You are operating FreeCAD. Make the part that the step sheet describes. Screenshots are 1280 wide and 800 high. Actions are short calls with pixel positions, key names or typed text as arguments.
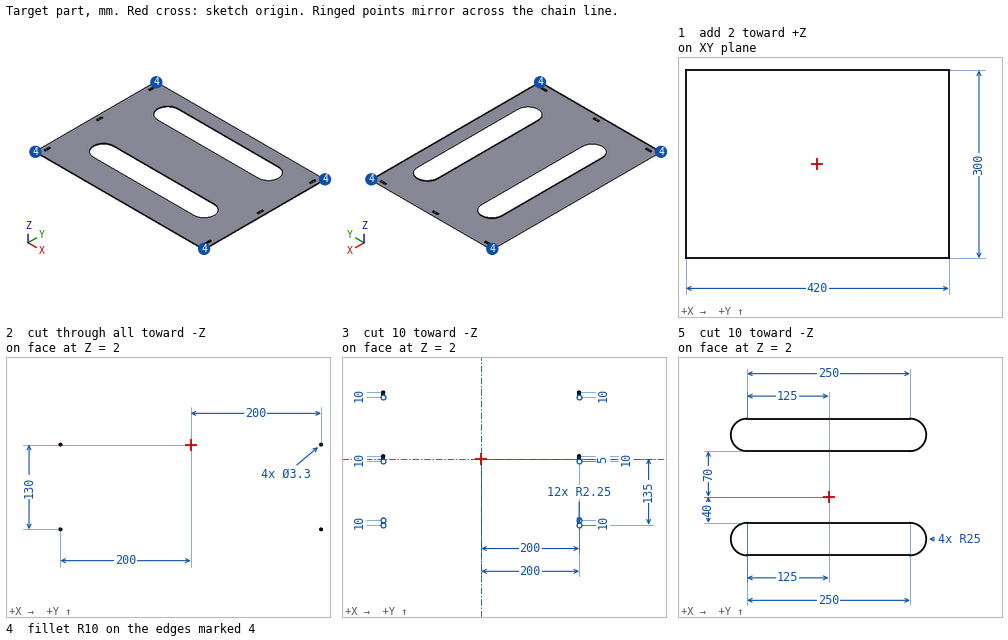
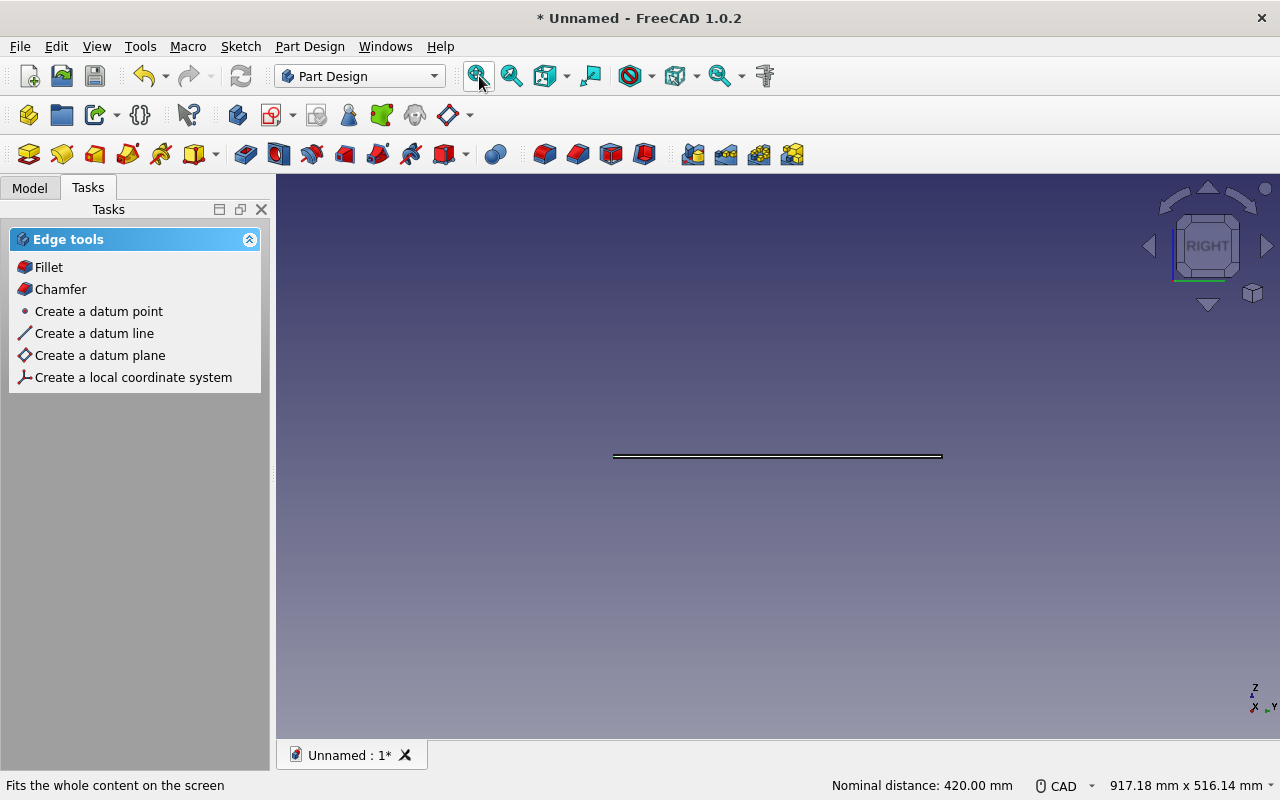
scroll(942, 455, up, 15)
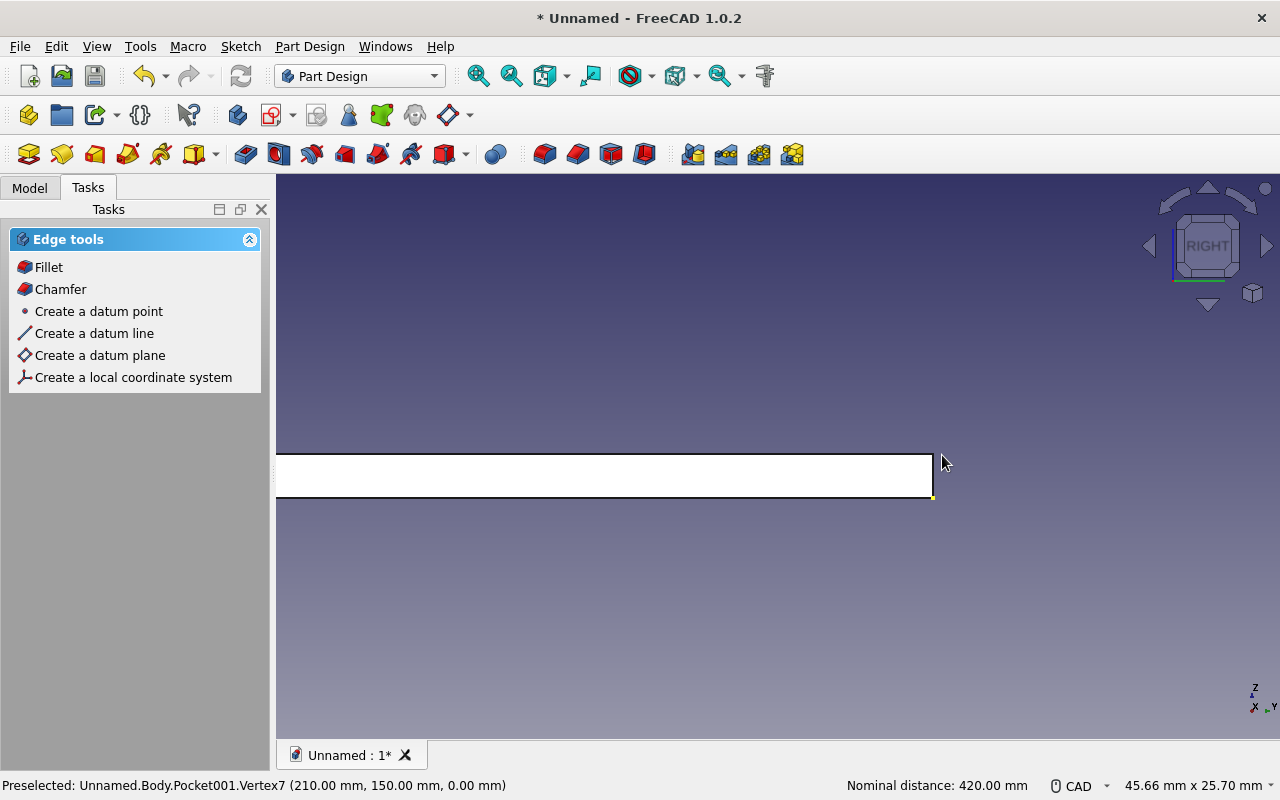
click(933, 475, ctrl)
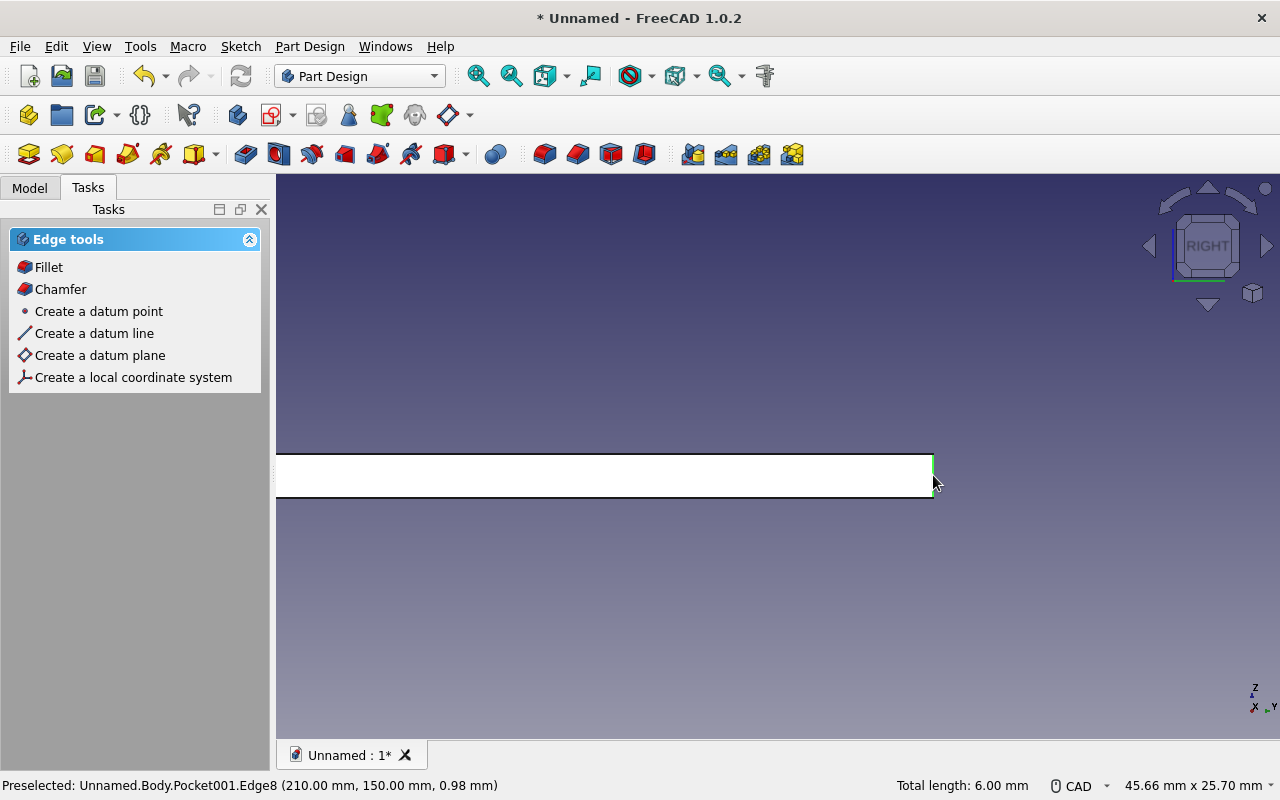
key(v)
key(f)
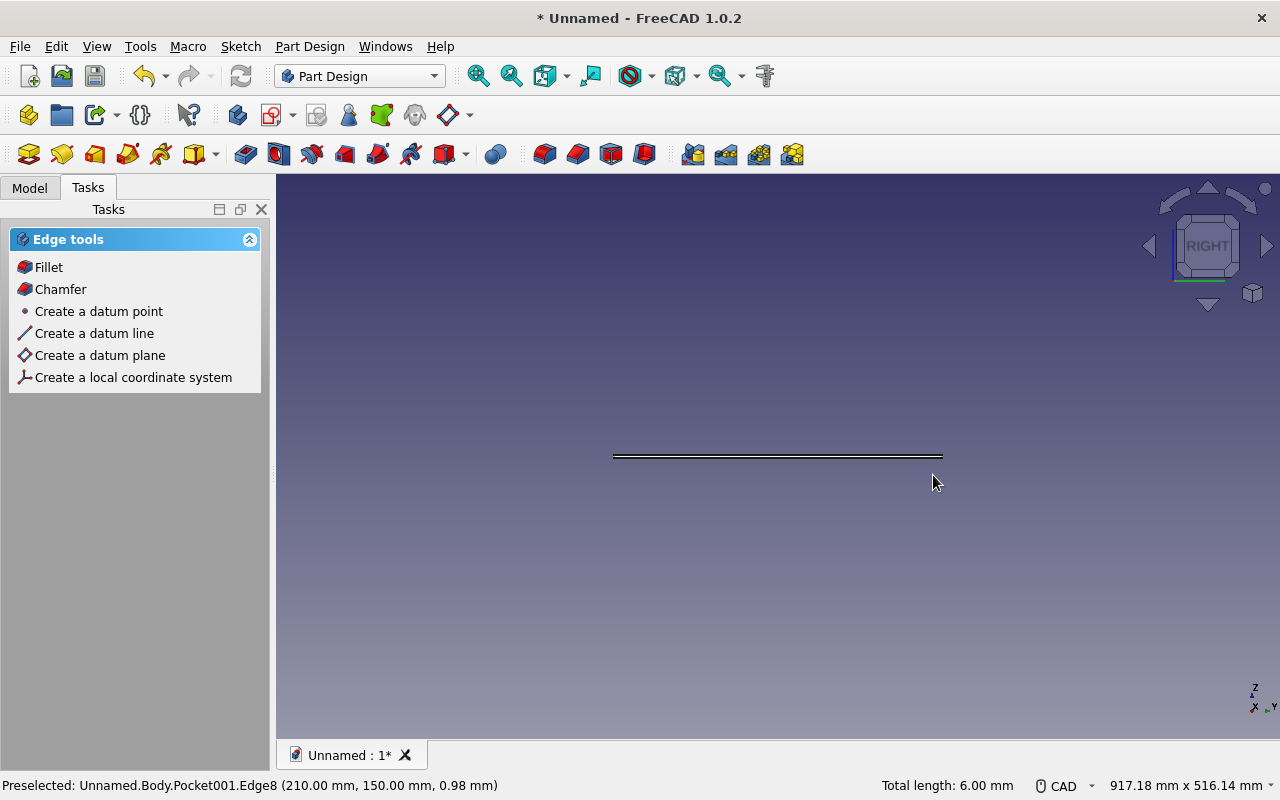
key(5)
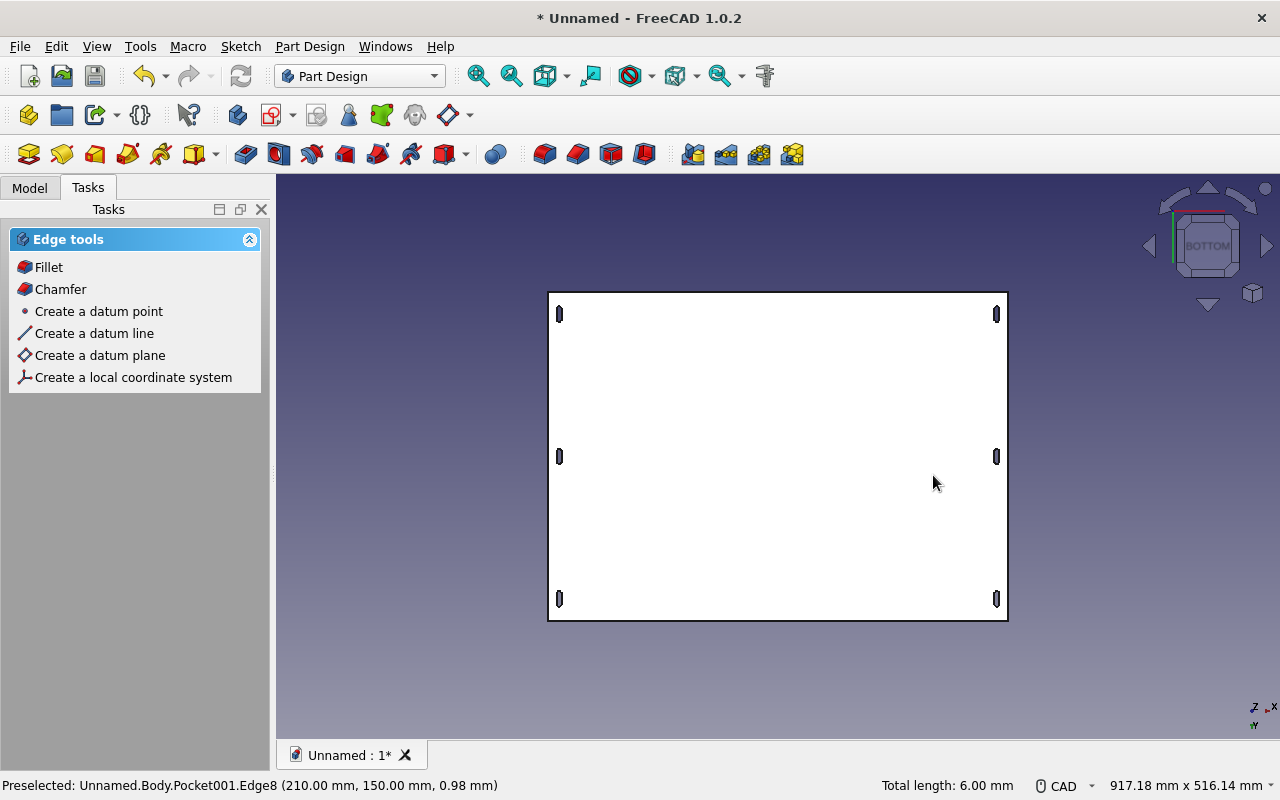
scroll(548, 620, up, 15)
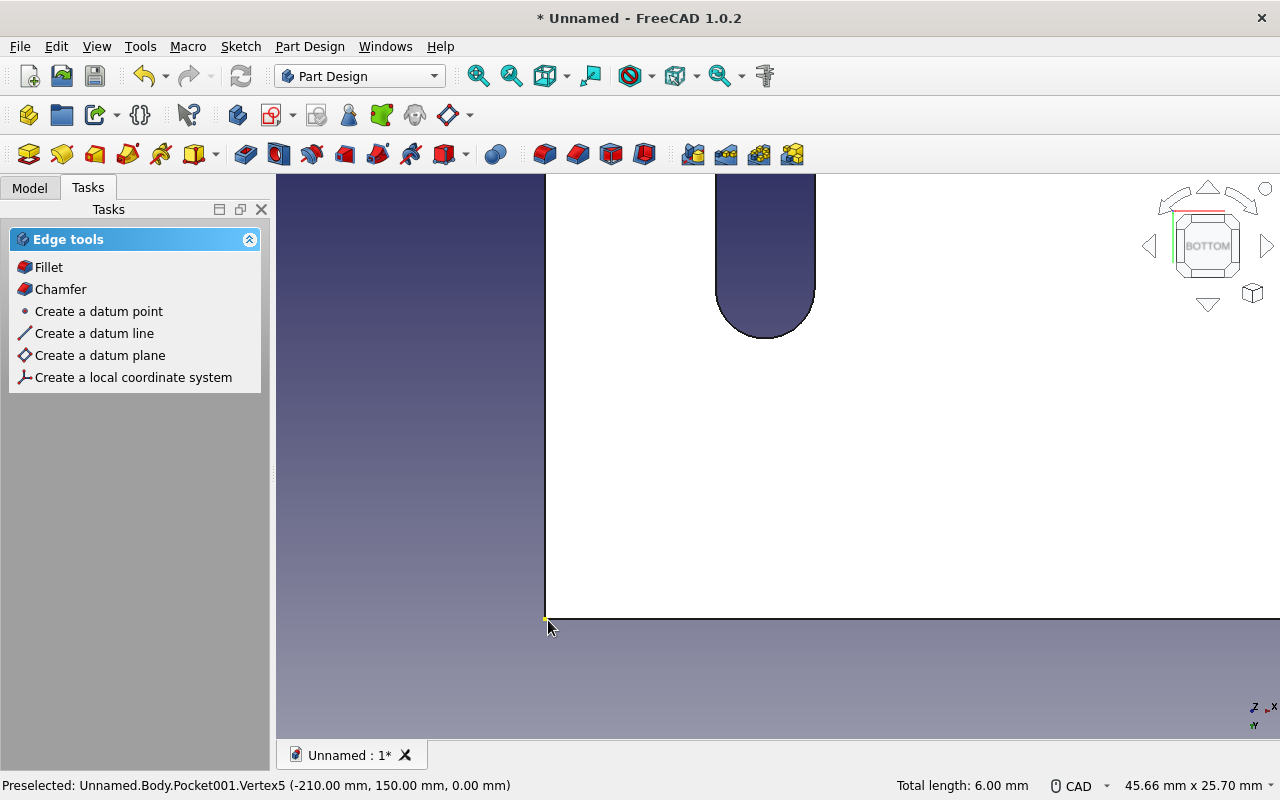
click(479, 76)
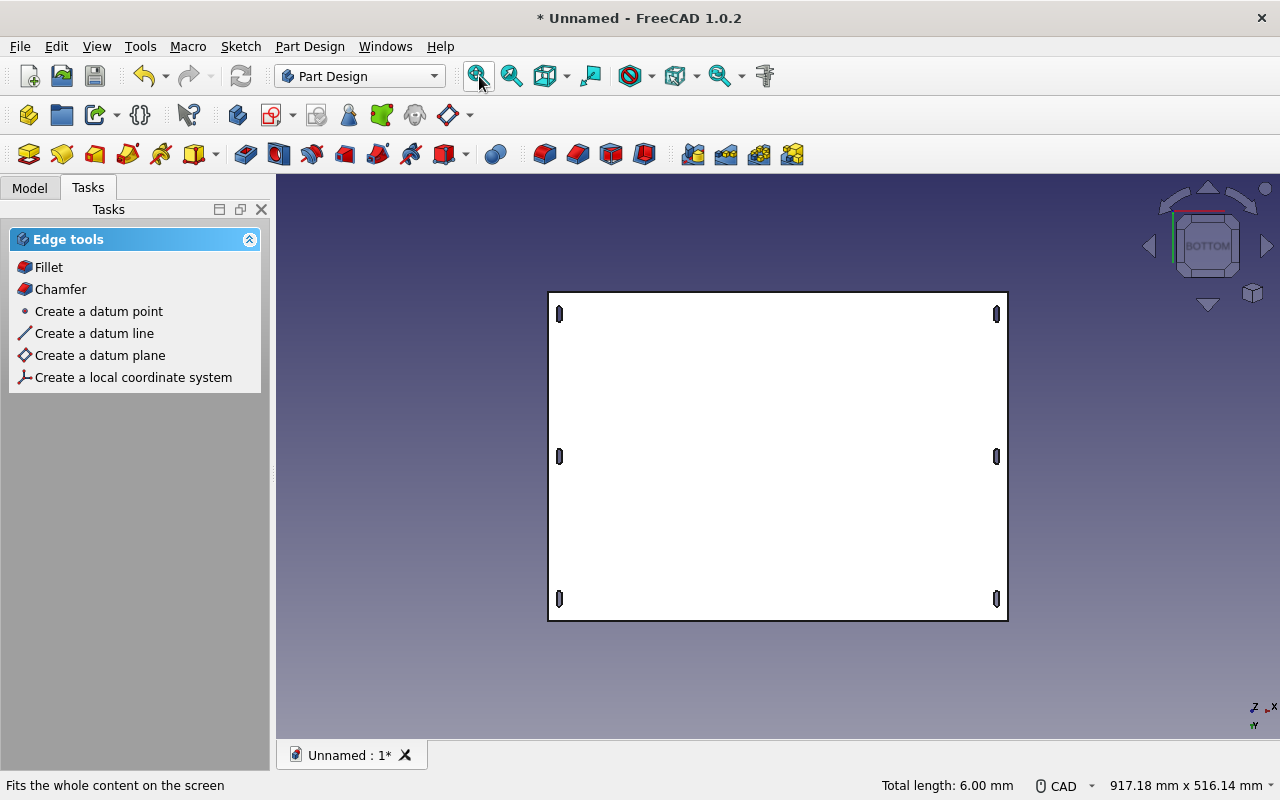
key(4)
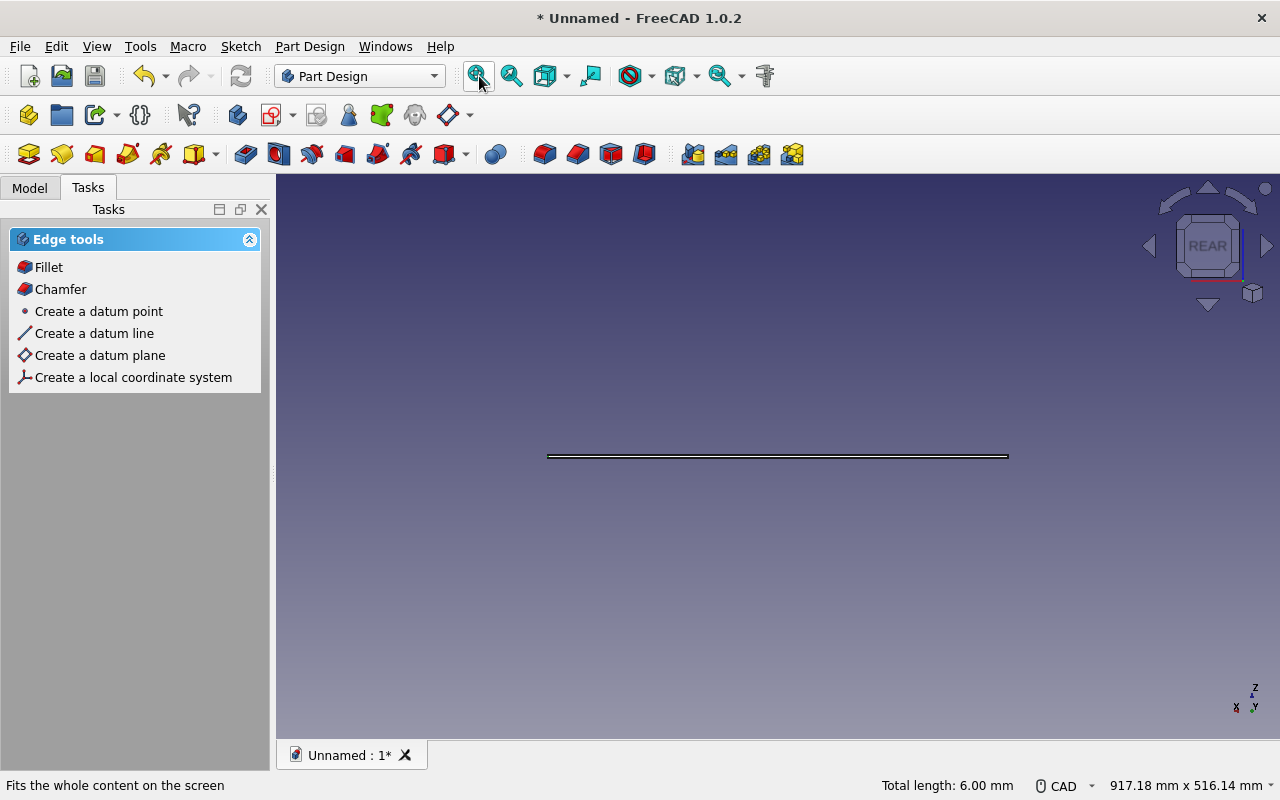
scroll(1008, 455, up, 15)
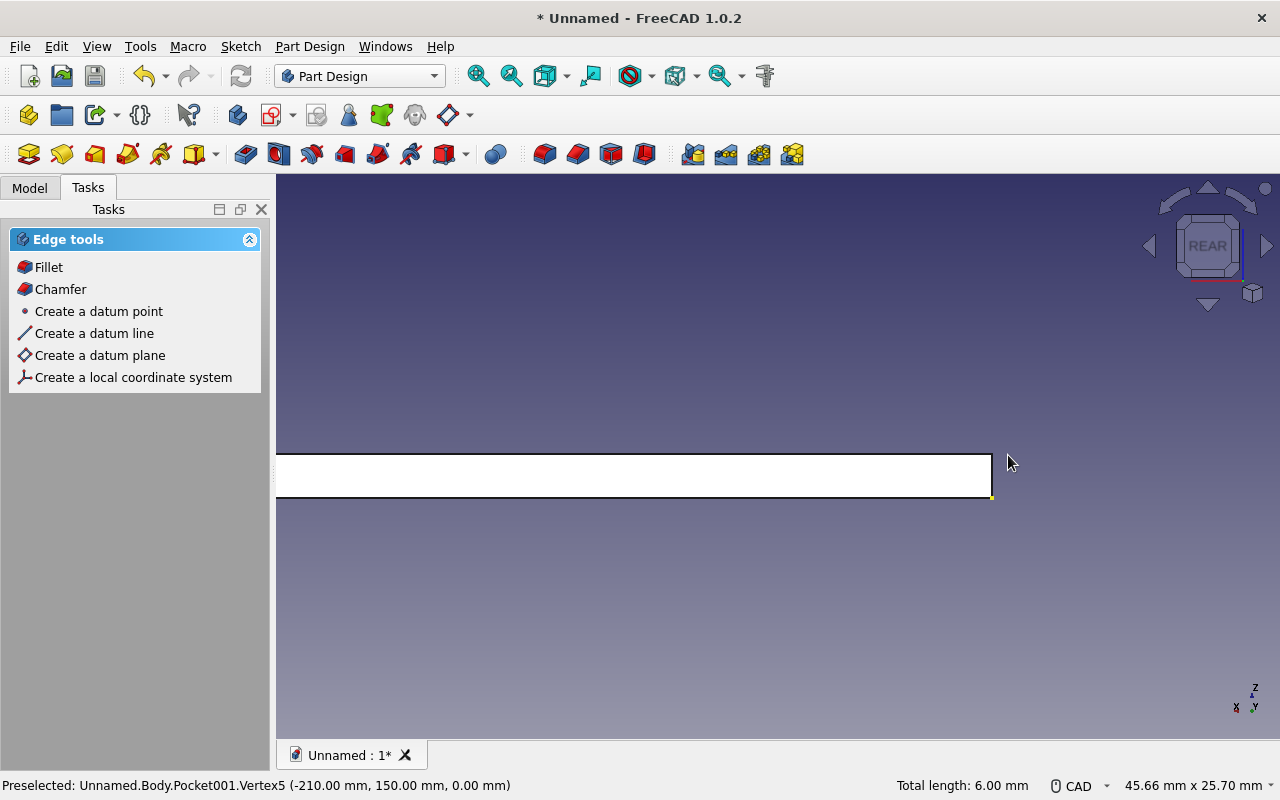
click(992, 475, ctrl)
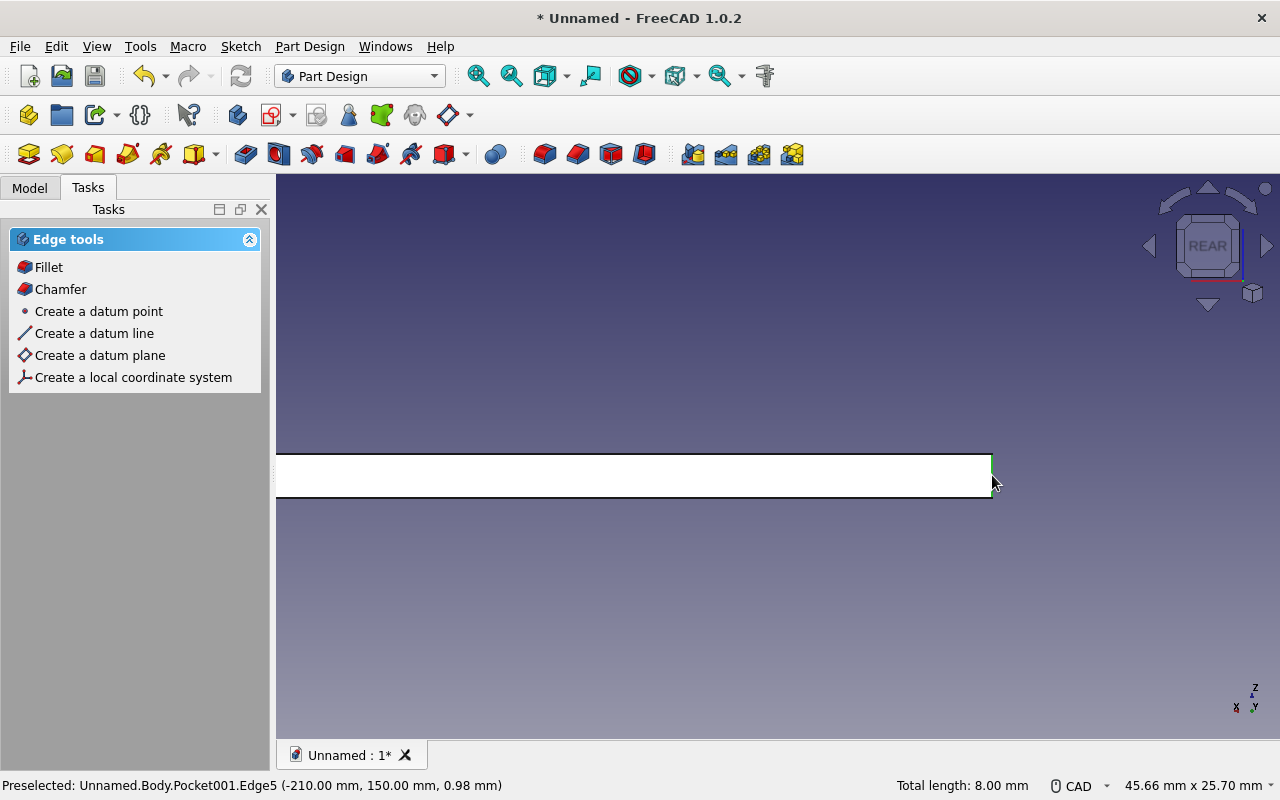
click(545, 154)